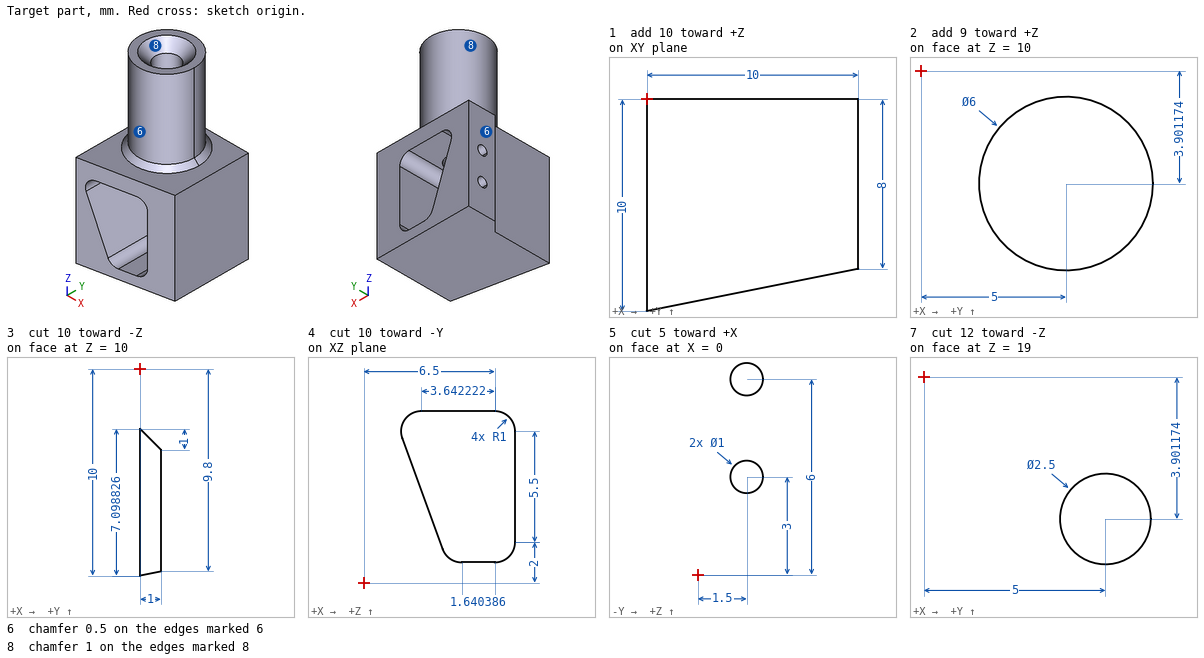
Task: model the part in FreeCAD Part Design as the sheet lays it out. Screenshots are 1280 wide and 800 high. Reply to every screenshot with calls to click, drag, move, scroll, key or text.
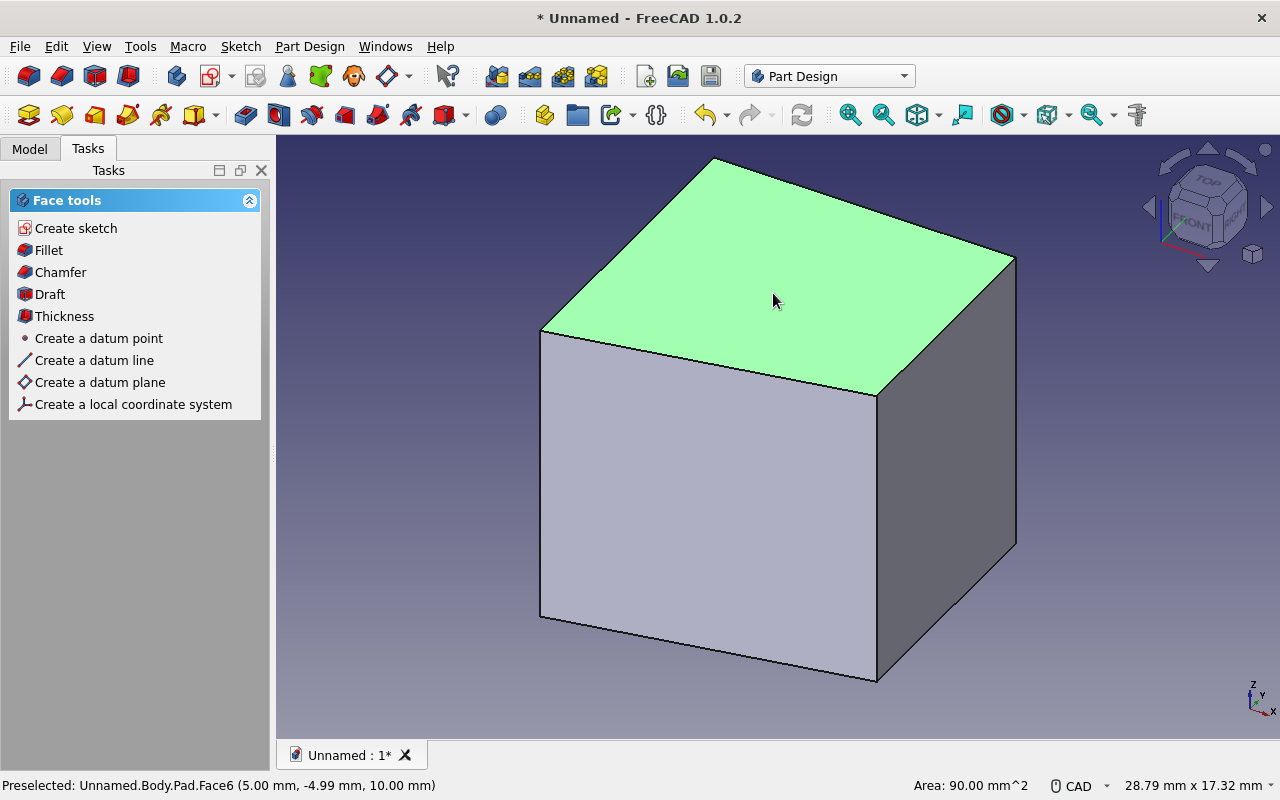
click(210, 76)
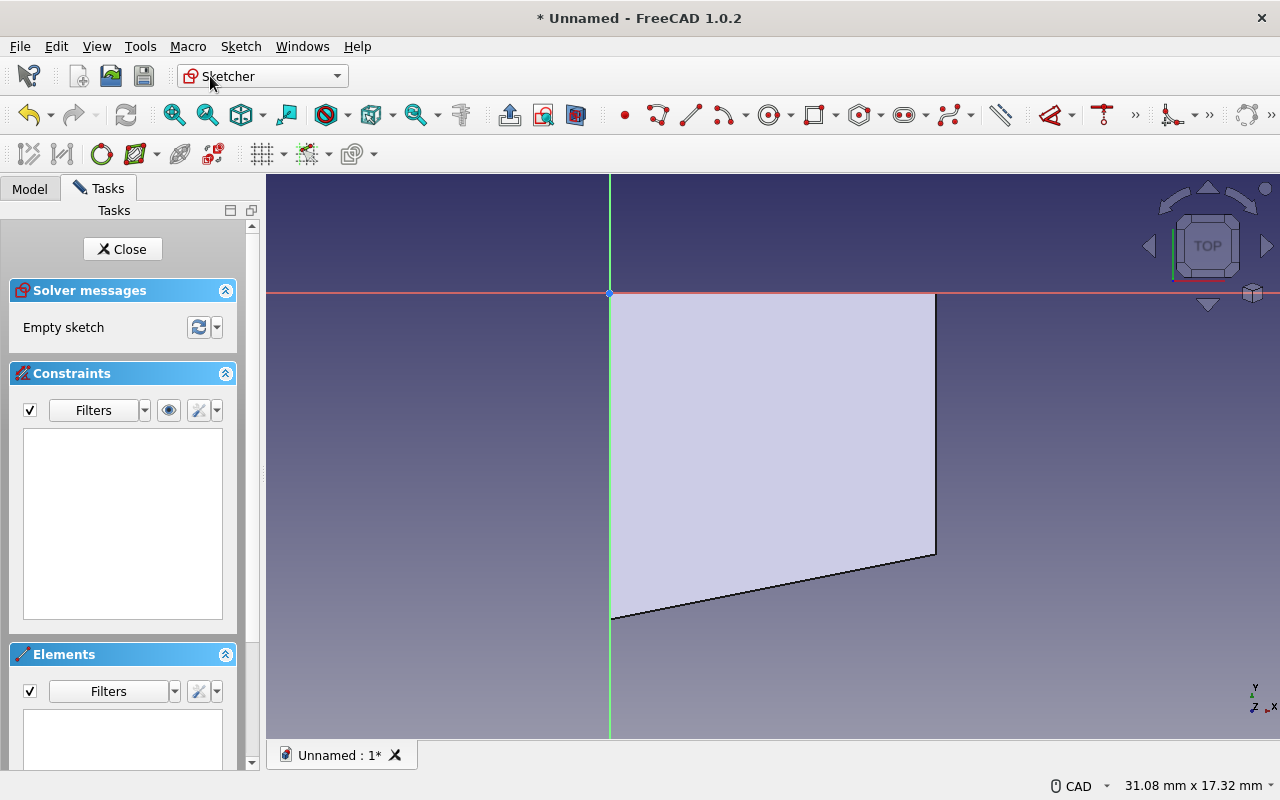
scroll(813, 303, up, 2)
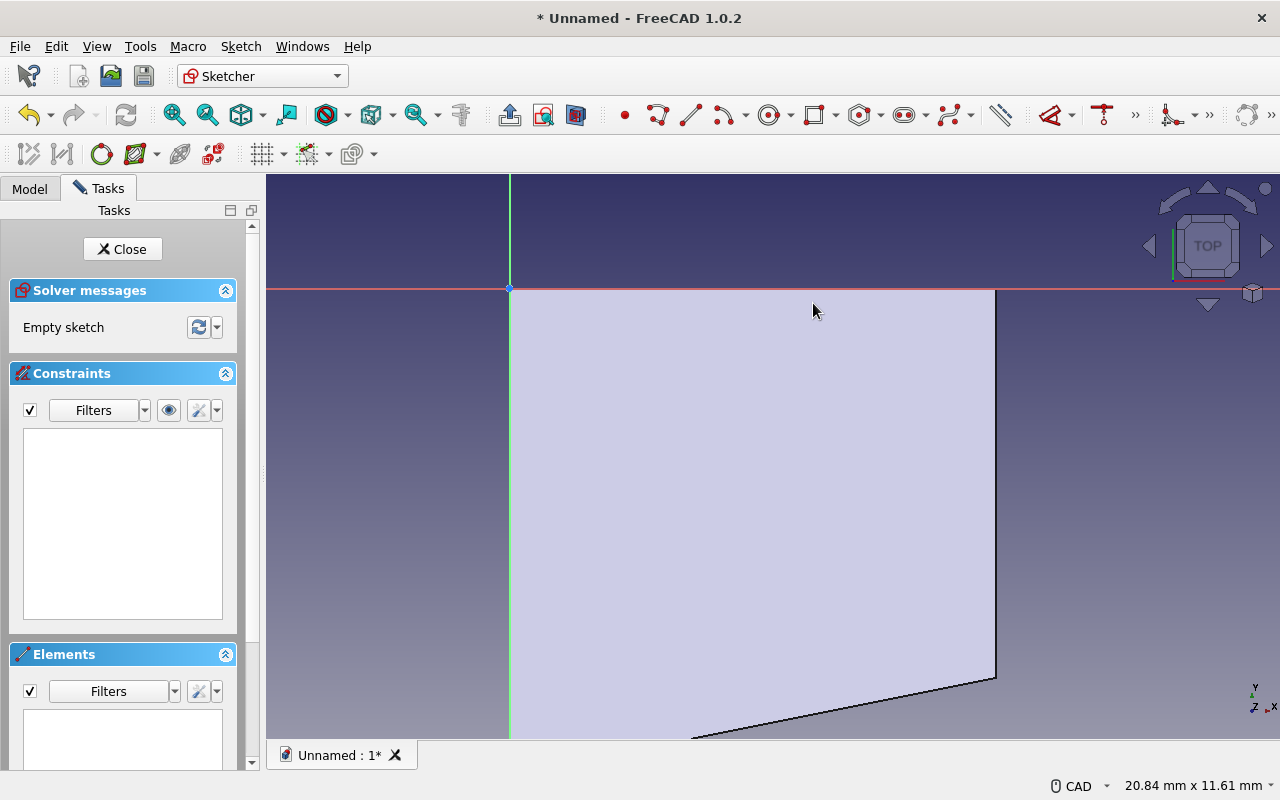
key(g)
key(c)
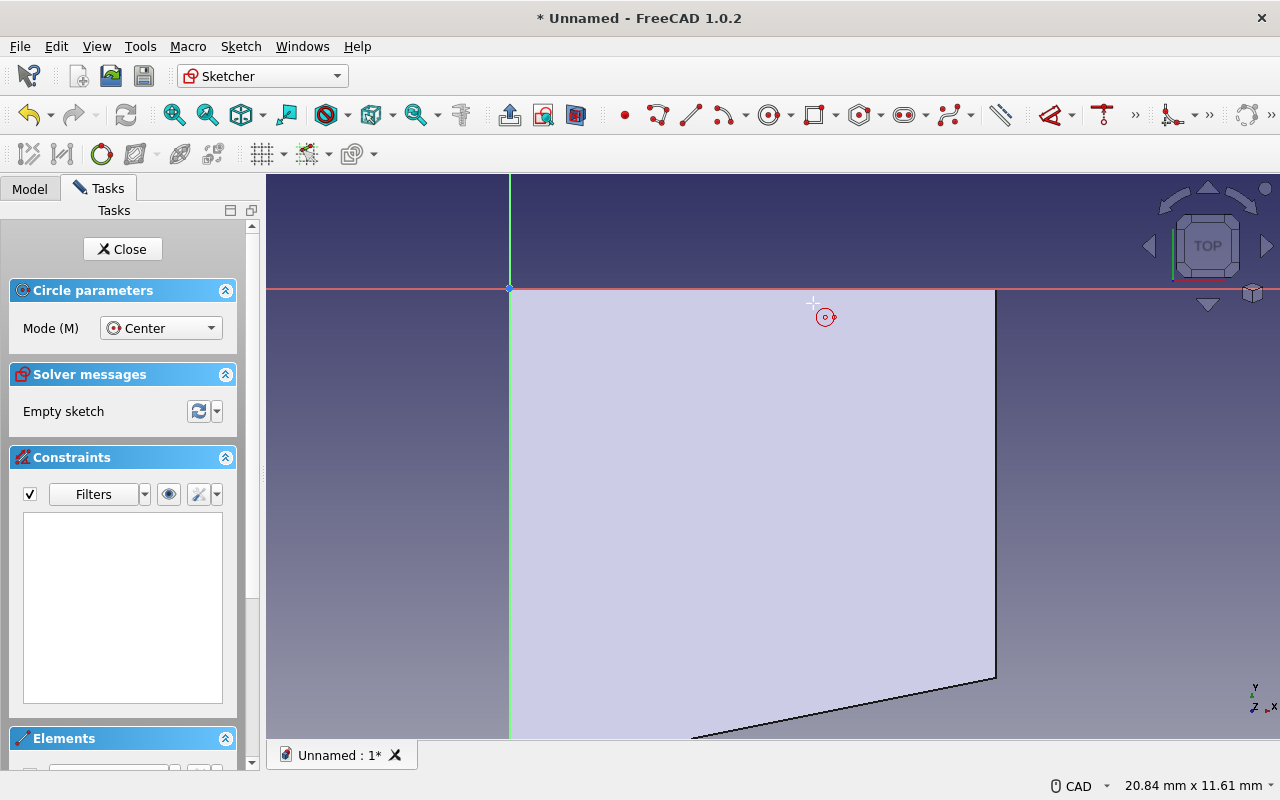
click(753, 478)
click(856, 375)
key(Escape)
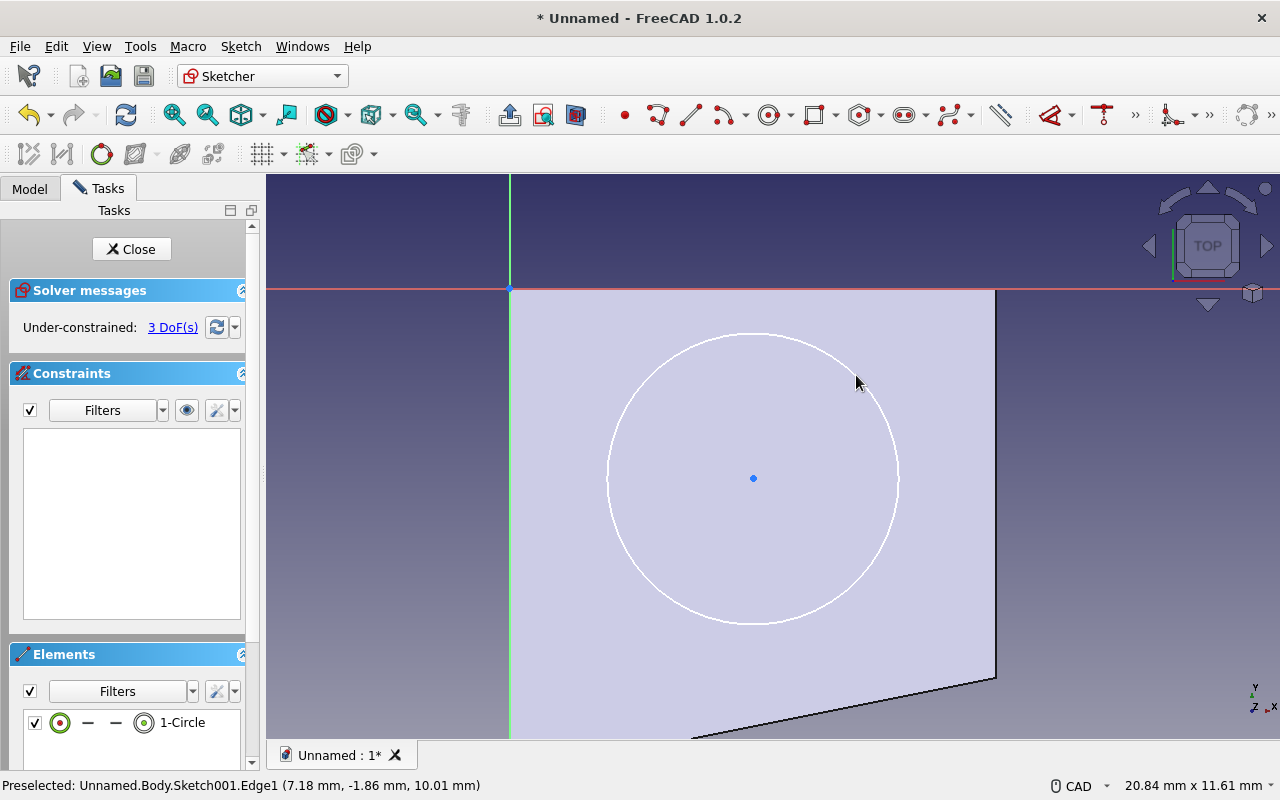
key(d)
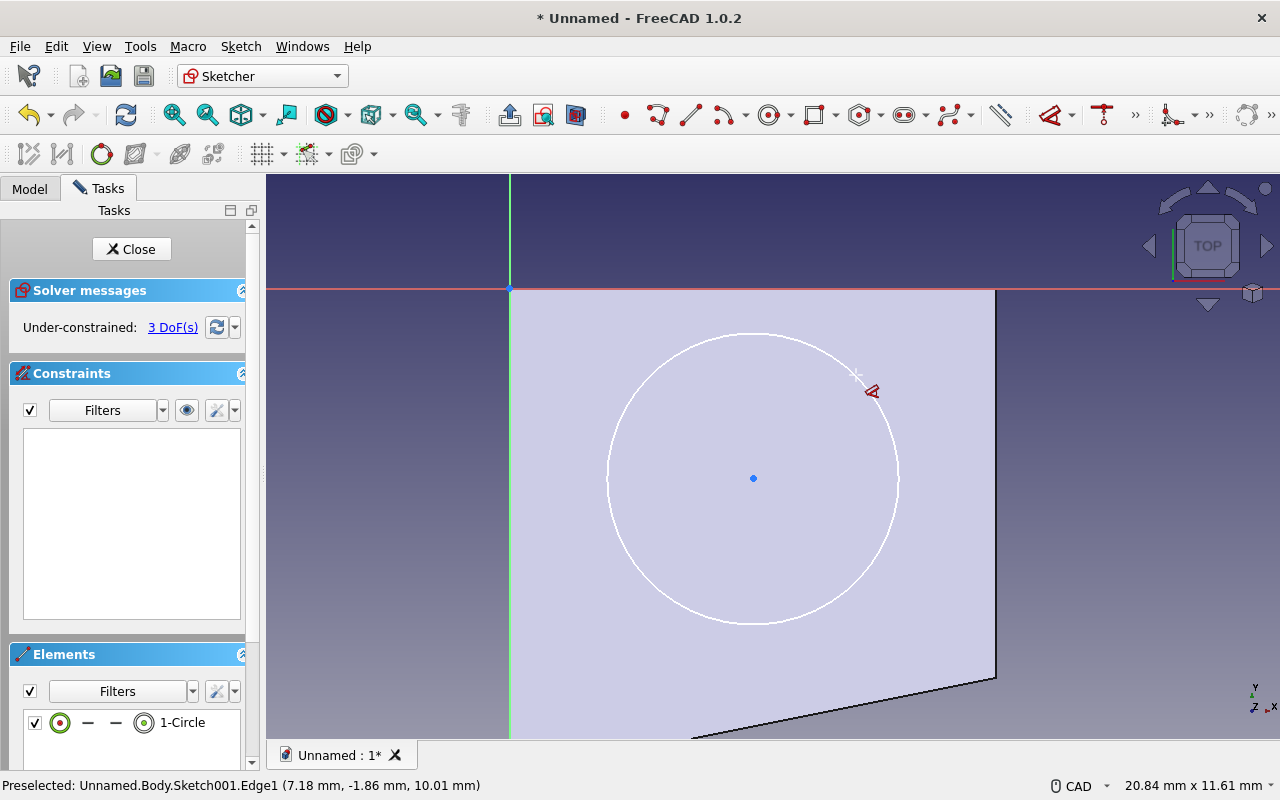
click(856, 376)
click(879, 353)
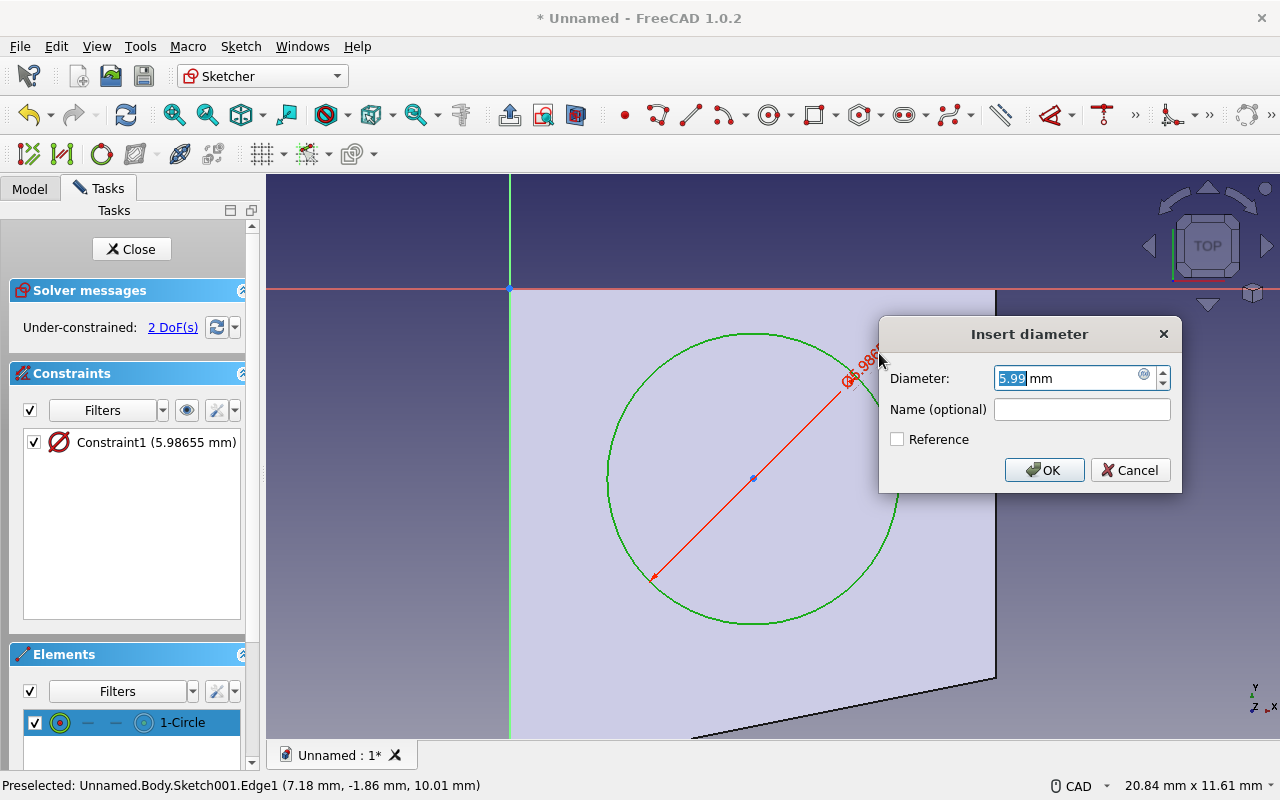
text(6)
key(Return)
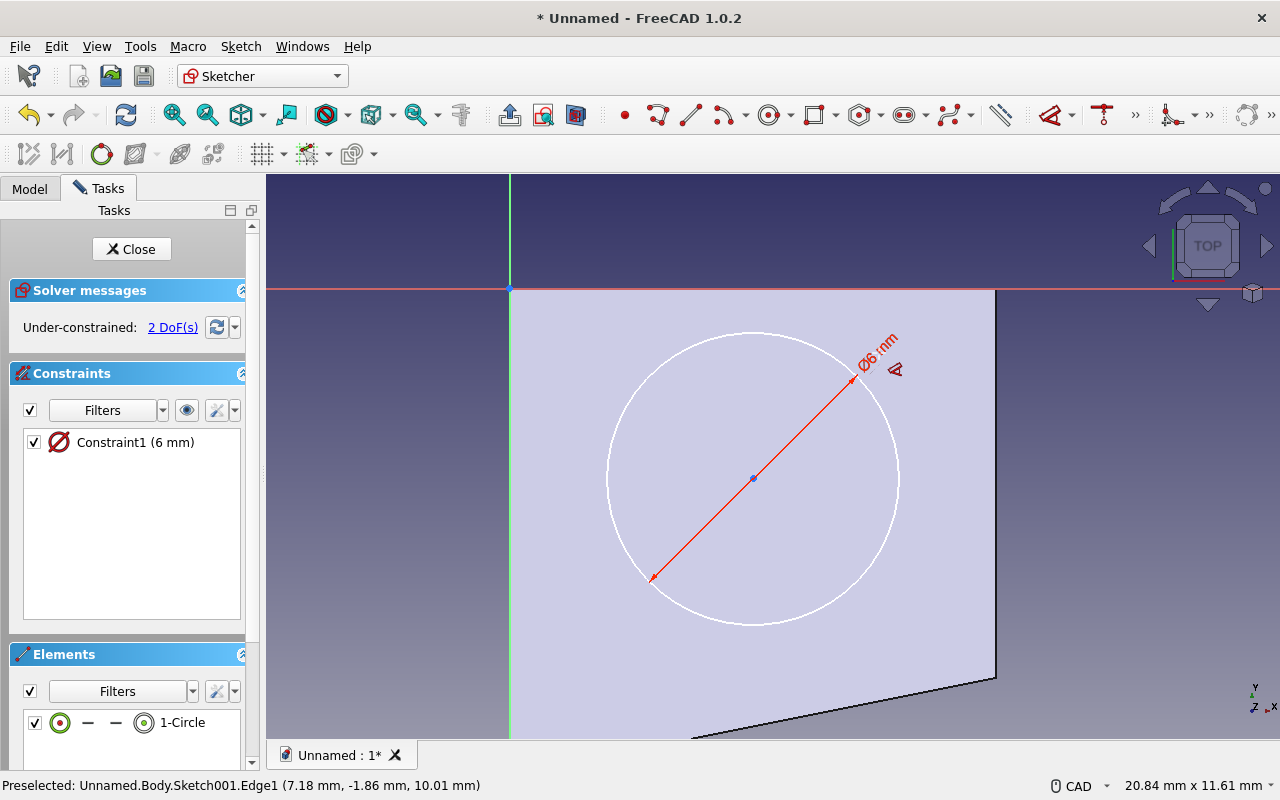
click(753, 479)
click(631, 255)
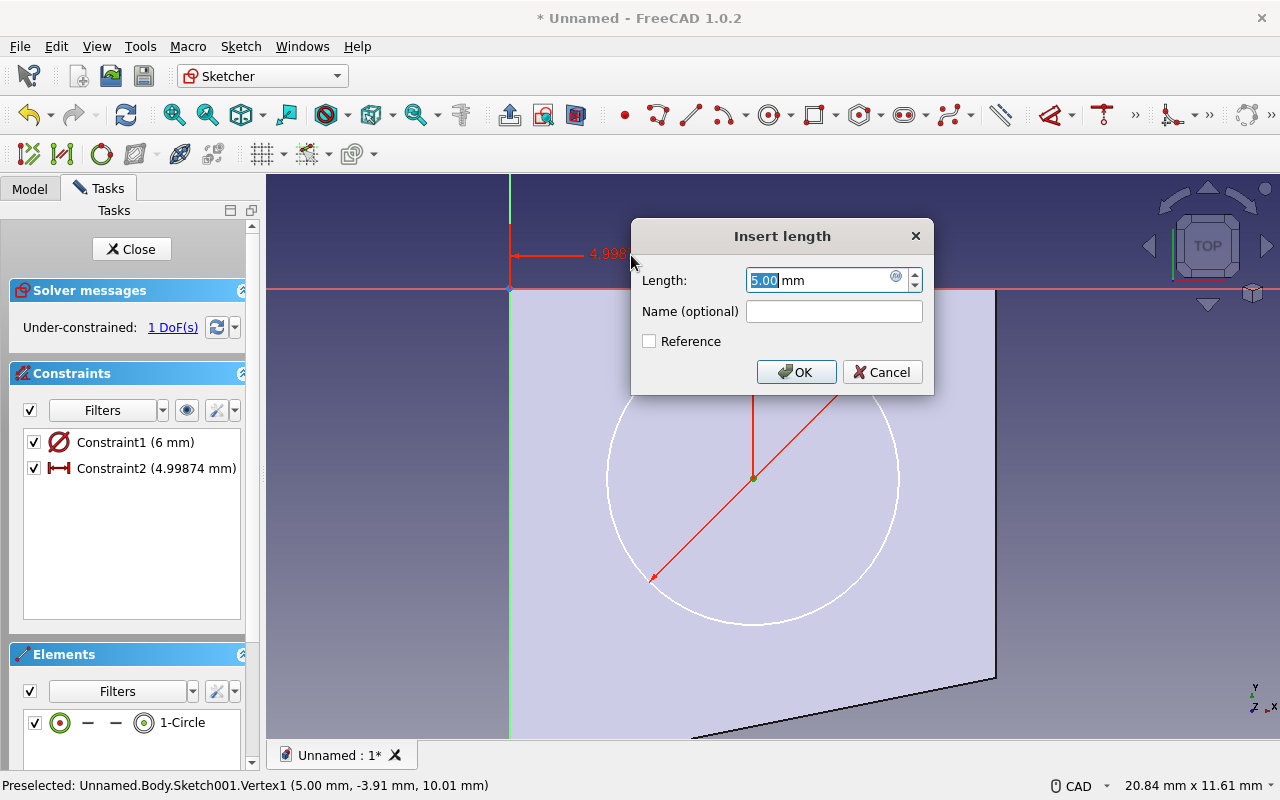
text(5)
key(Return)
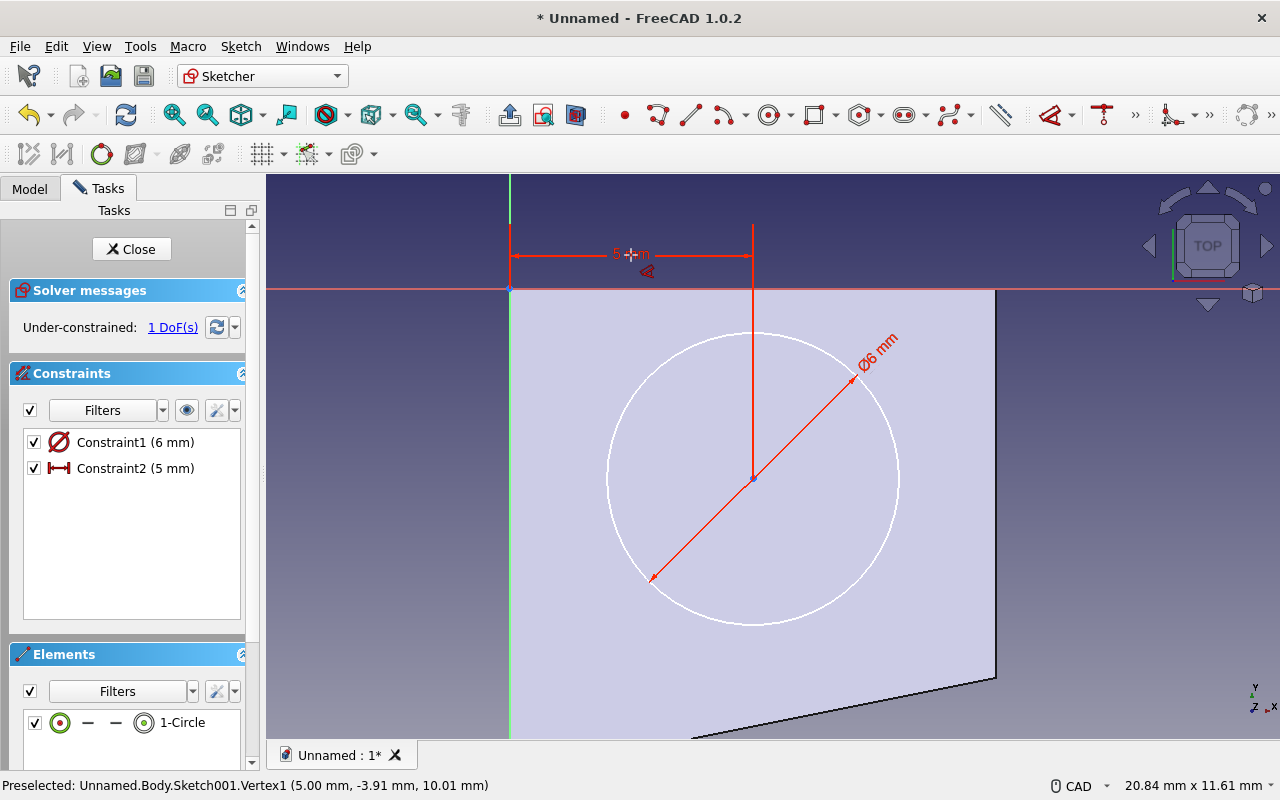
click(753, 479)
click(476, 384)